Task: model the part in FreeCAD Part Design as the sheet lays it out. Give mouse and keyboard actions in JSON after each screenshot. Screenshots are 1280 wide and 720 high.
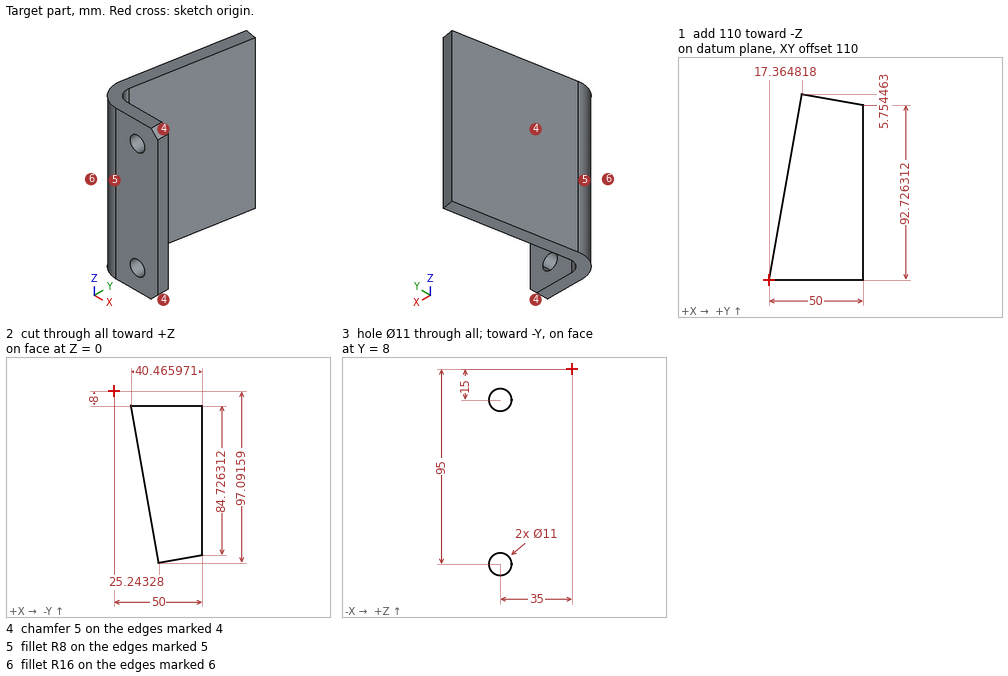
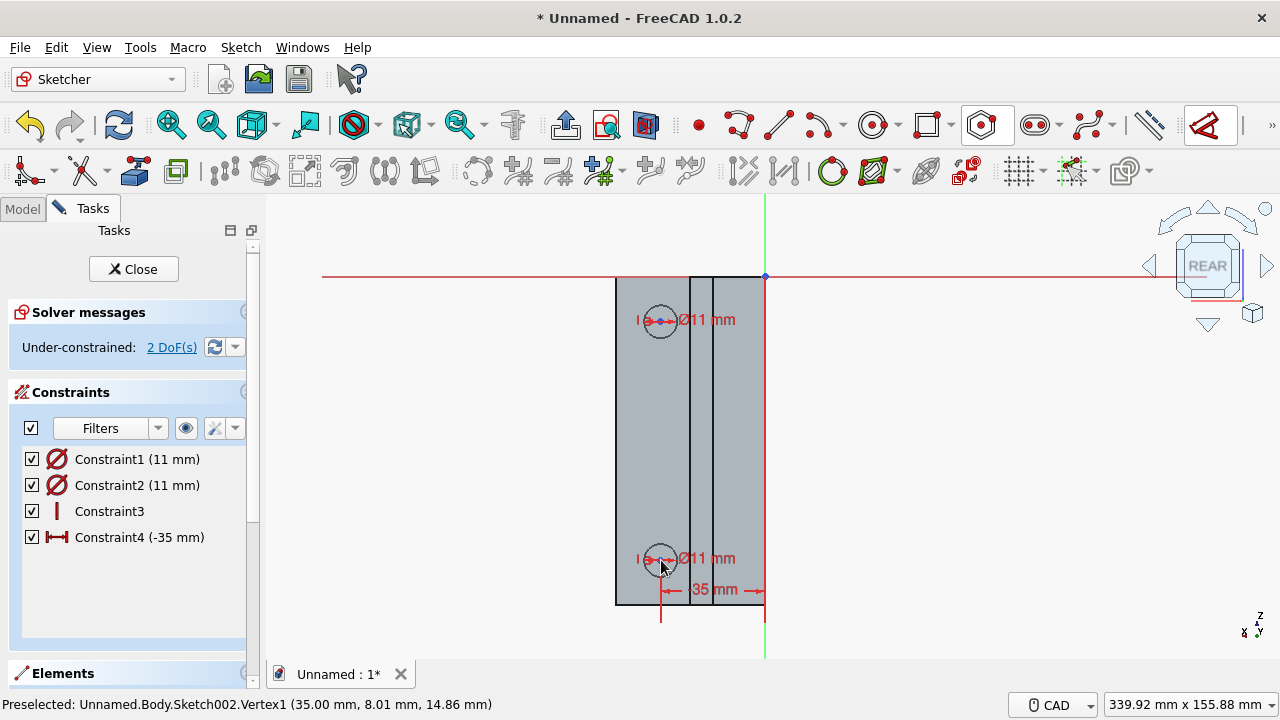
{"action": "left_click", "coordinate": [661, 560]}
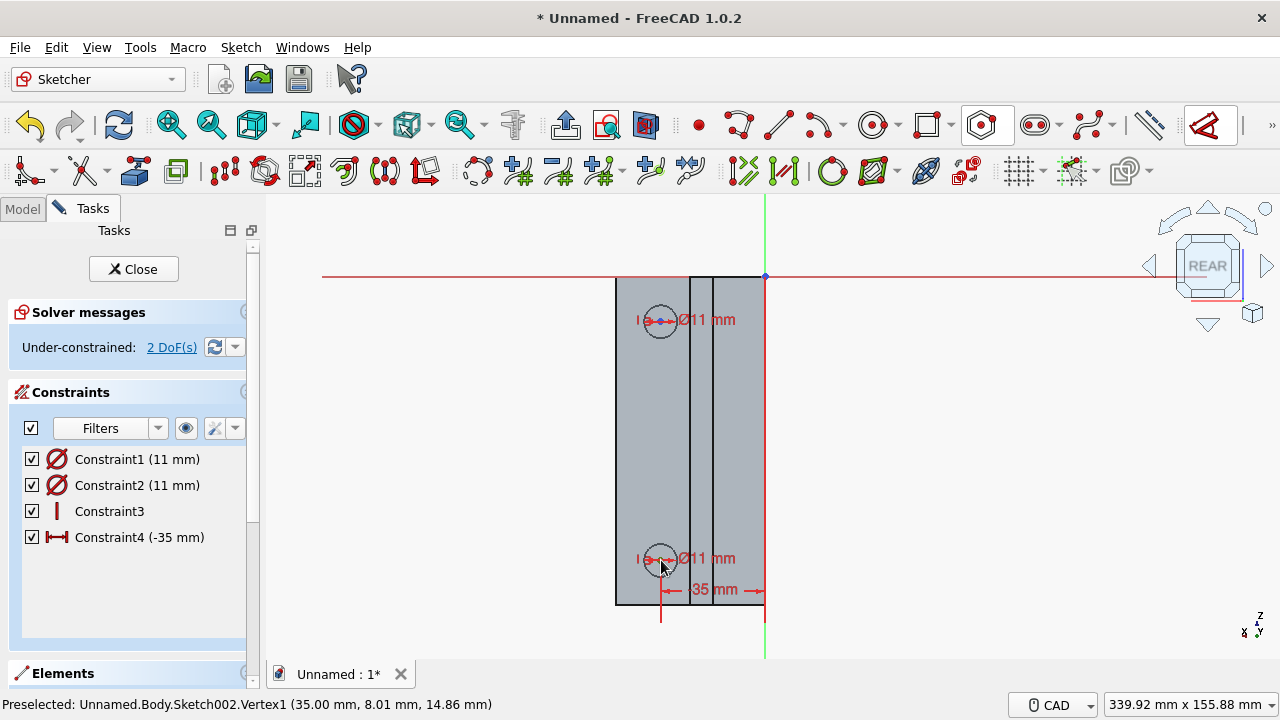
{"action": "key", "text": "i"}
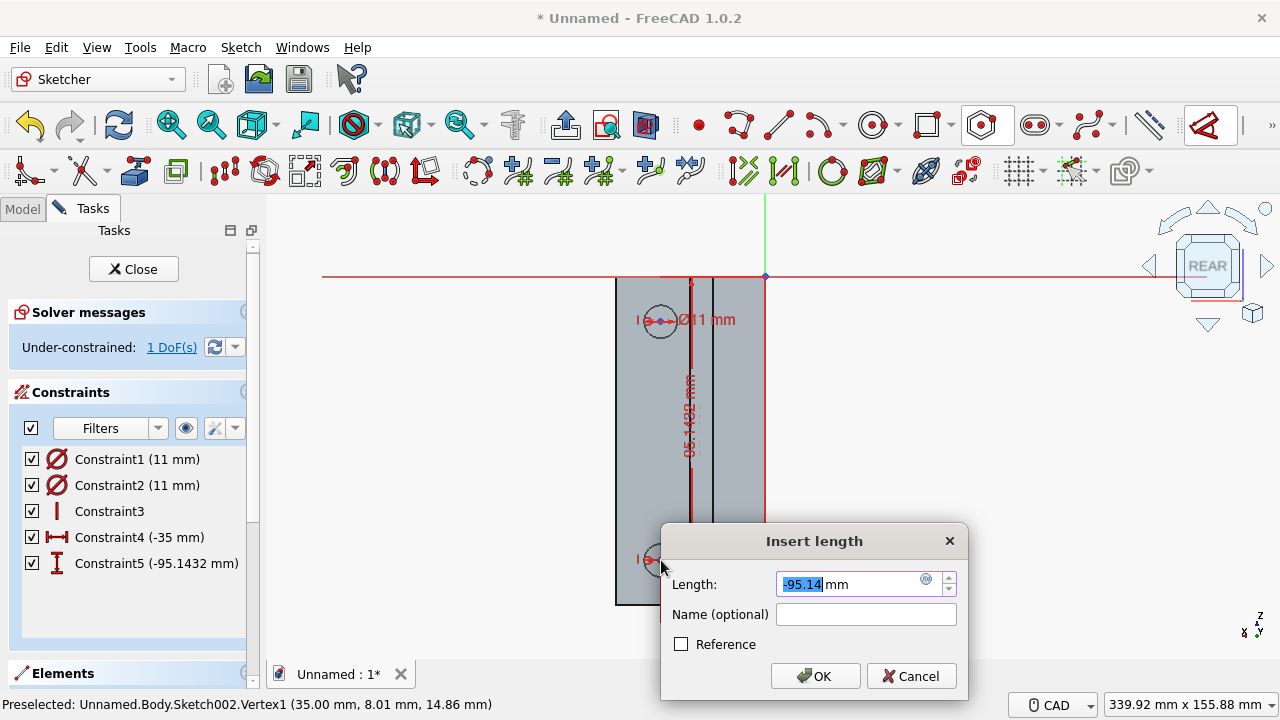
{"action": "type", "text": "-95"}
{"action": "key", "text": "Return"}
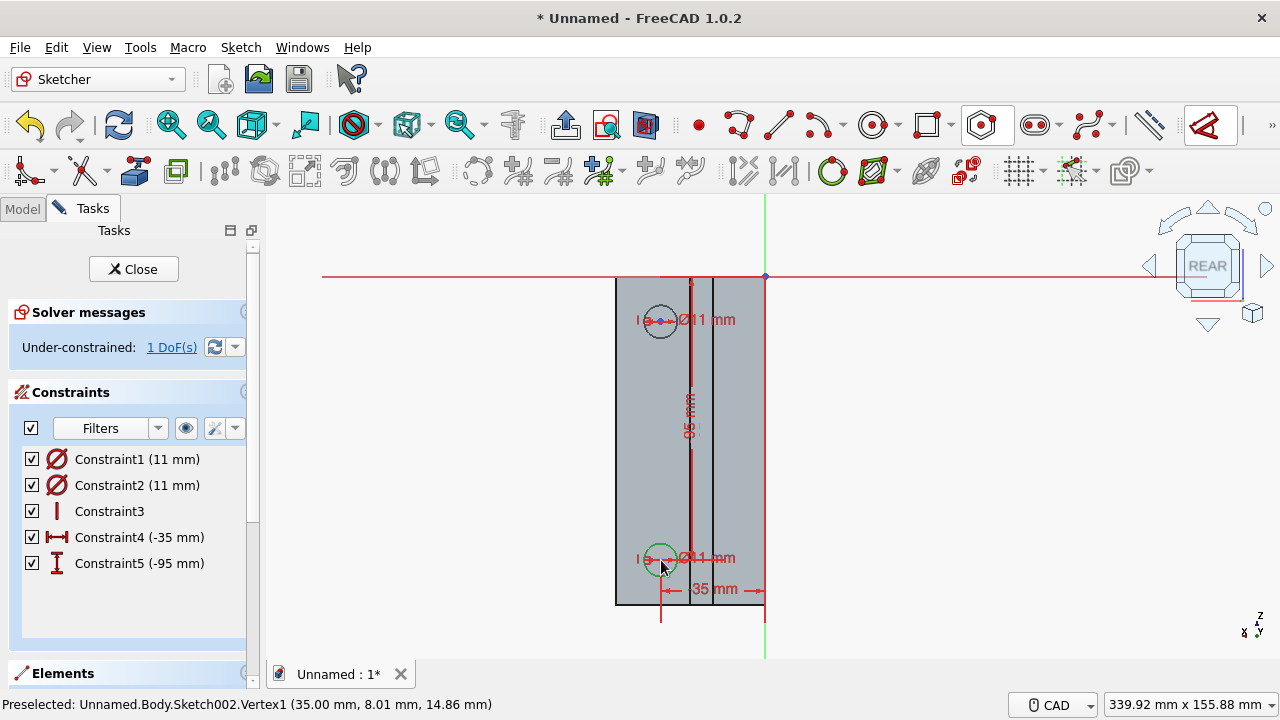
{"action": "left_click", "coordinate": [661, 322]}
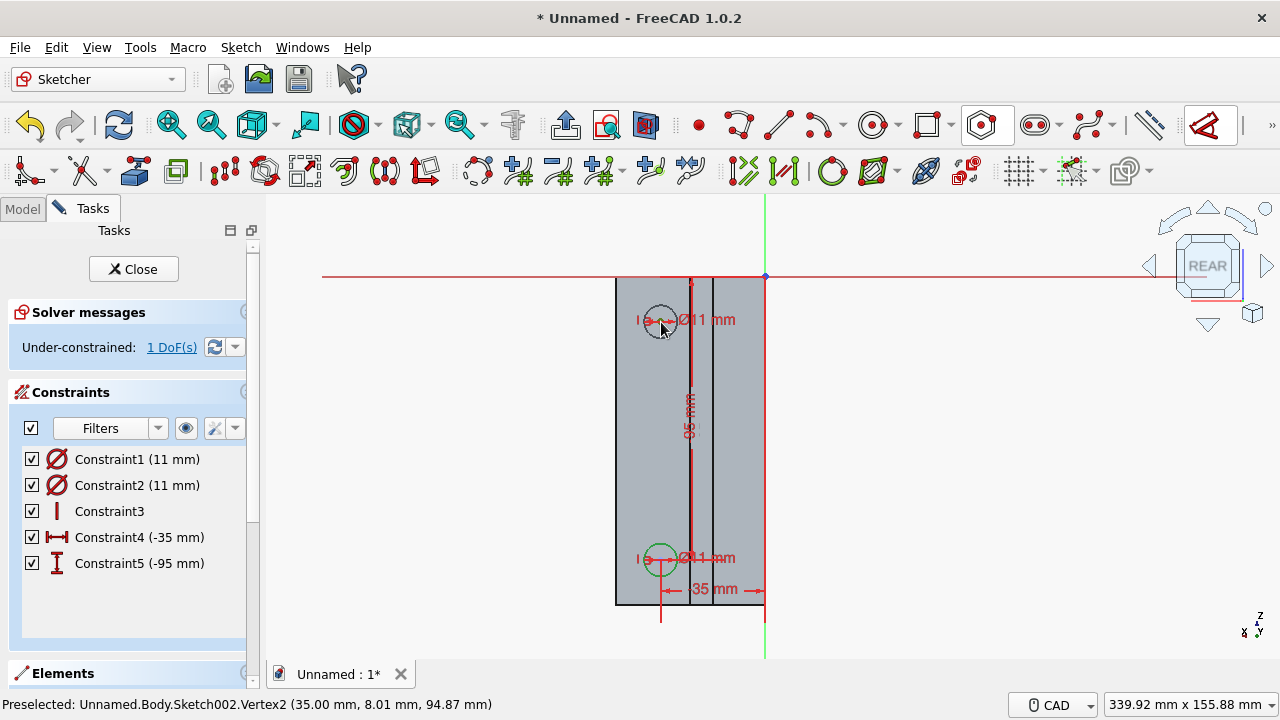
{"action": "left_click", "coordinate": [1232, 126]}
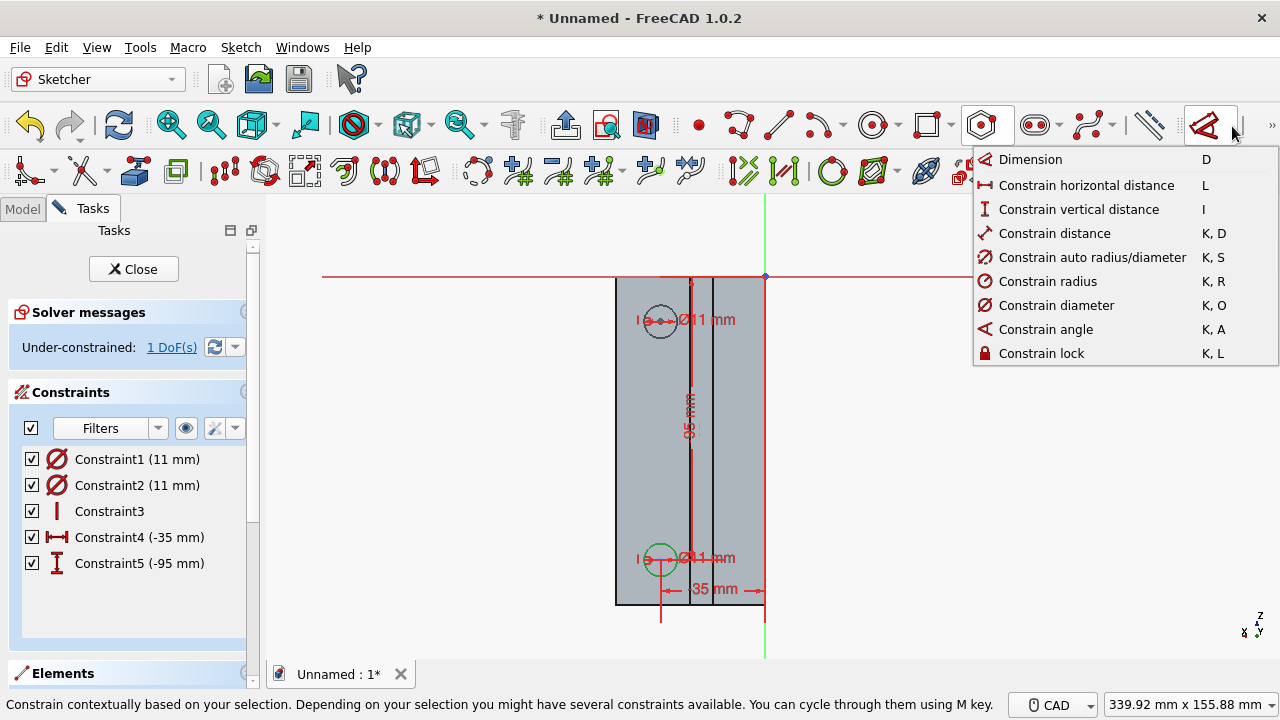
{"action": "left_click", "coordinate": [1126, 209]}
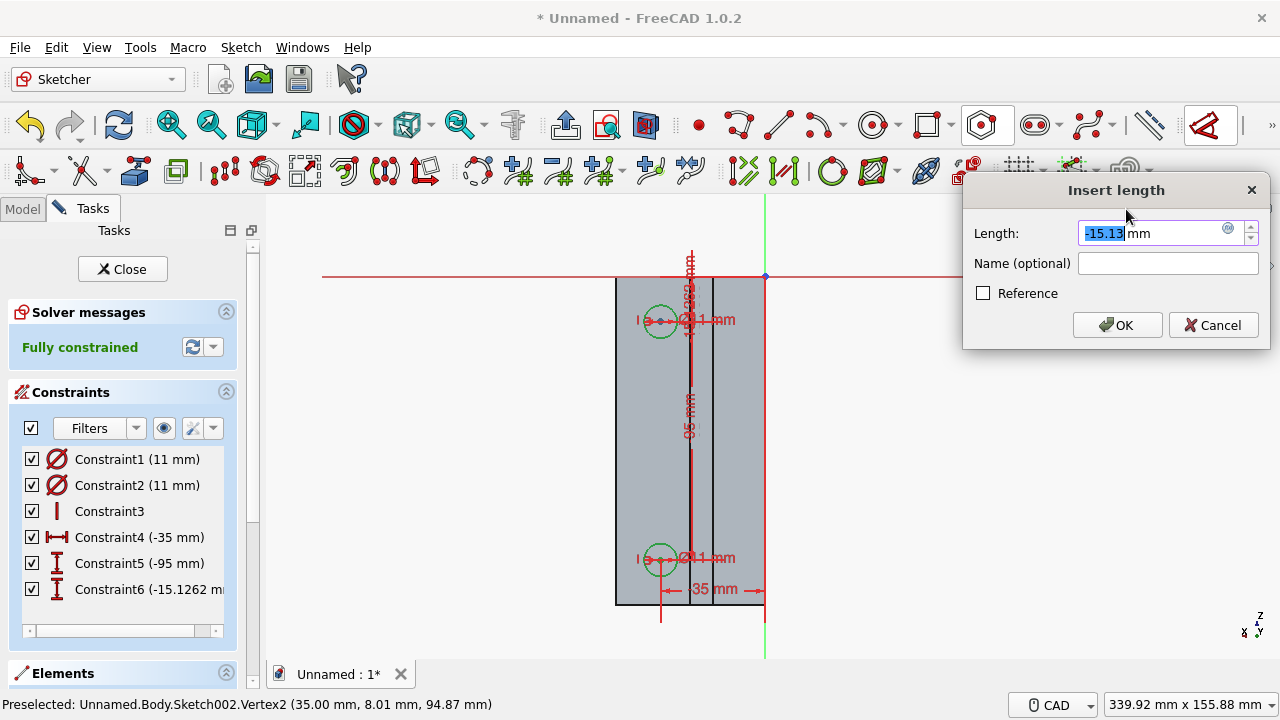
{"action": "type", "text": "-15"}
{"action": "key", "text": "Return"}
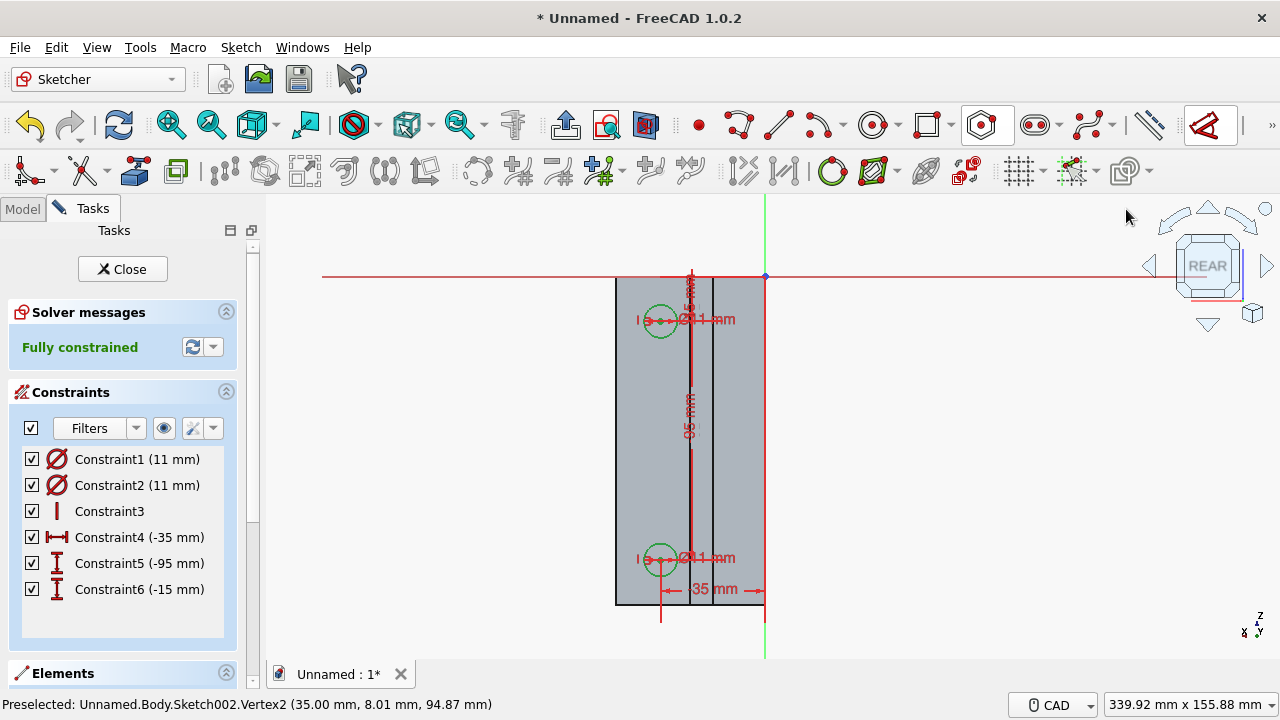
{"action": "left_click", "coordinate": [123, 269]}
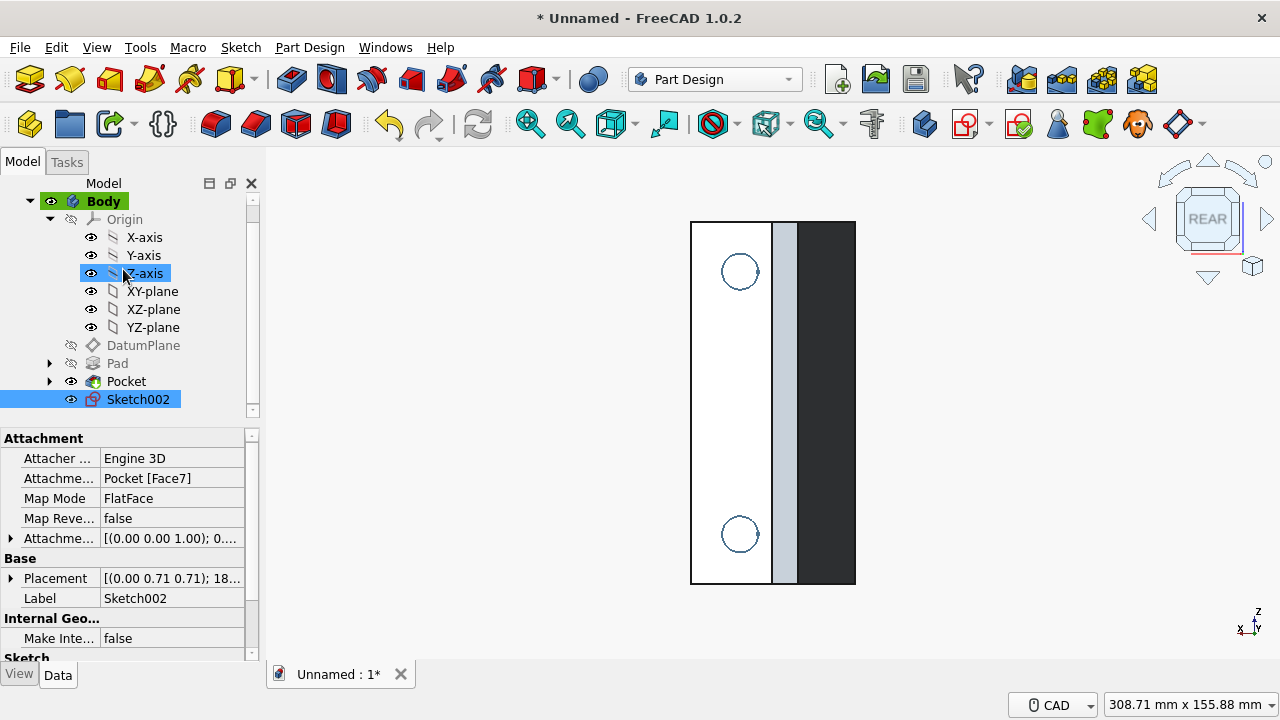
{"action": "left_click", "coordinate": [332, 80]}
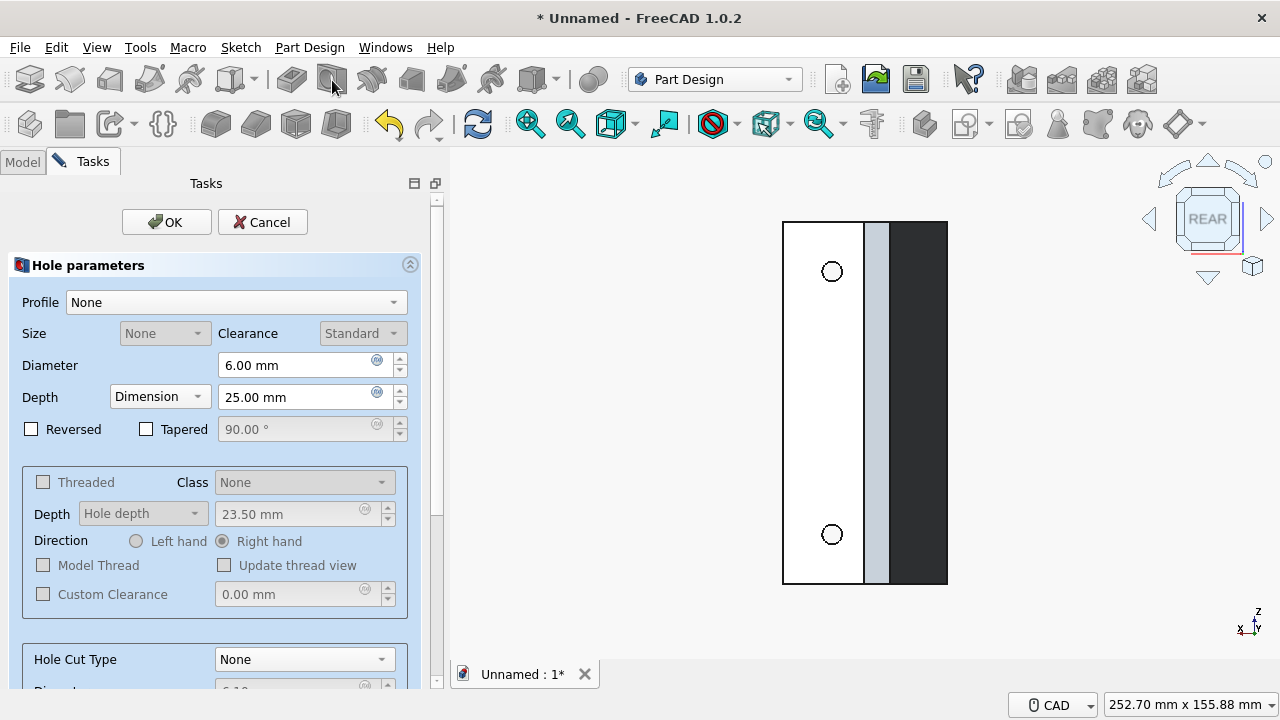
{"action": "triple_click", "coordinate": [305, 365]}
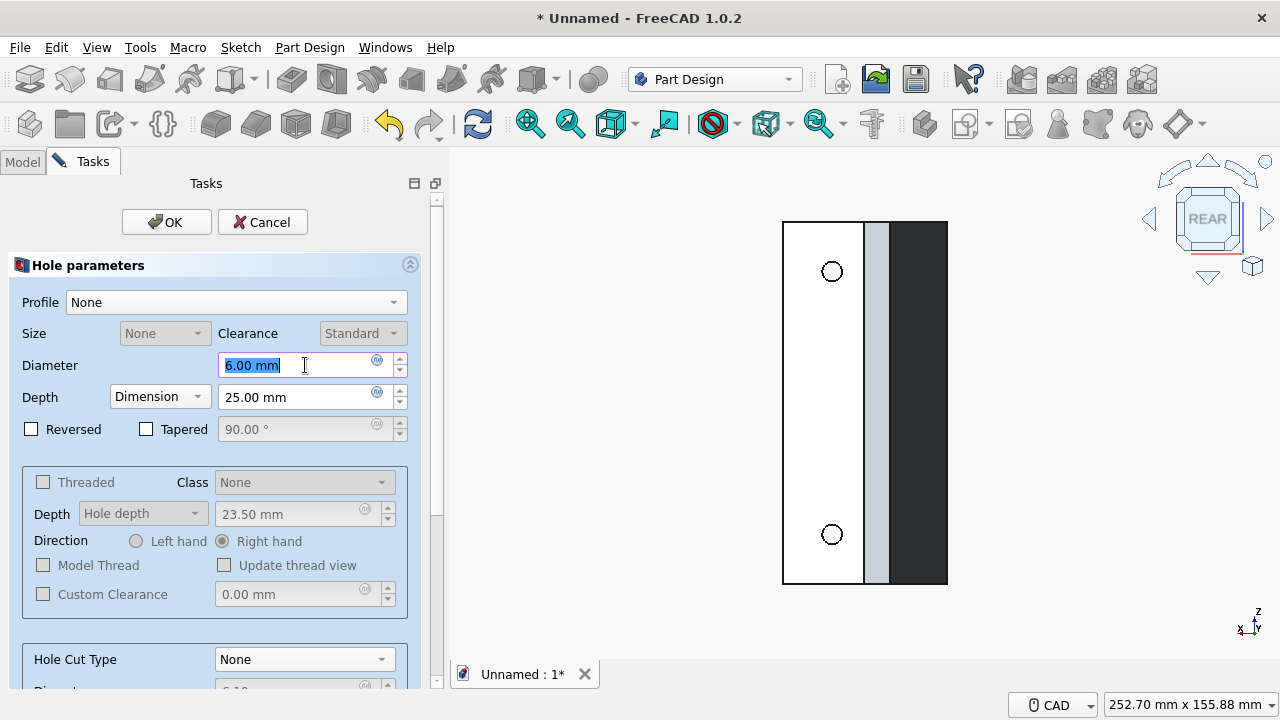
{"action": "type", "text": "11"}
{"action": "key", "text": "Tab"}